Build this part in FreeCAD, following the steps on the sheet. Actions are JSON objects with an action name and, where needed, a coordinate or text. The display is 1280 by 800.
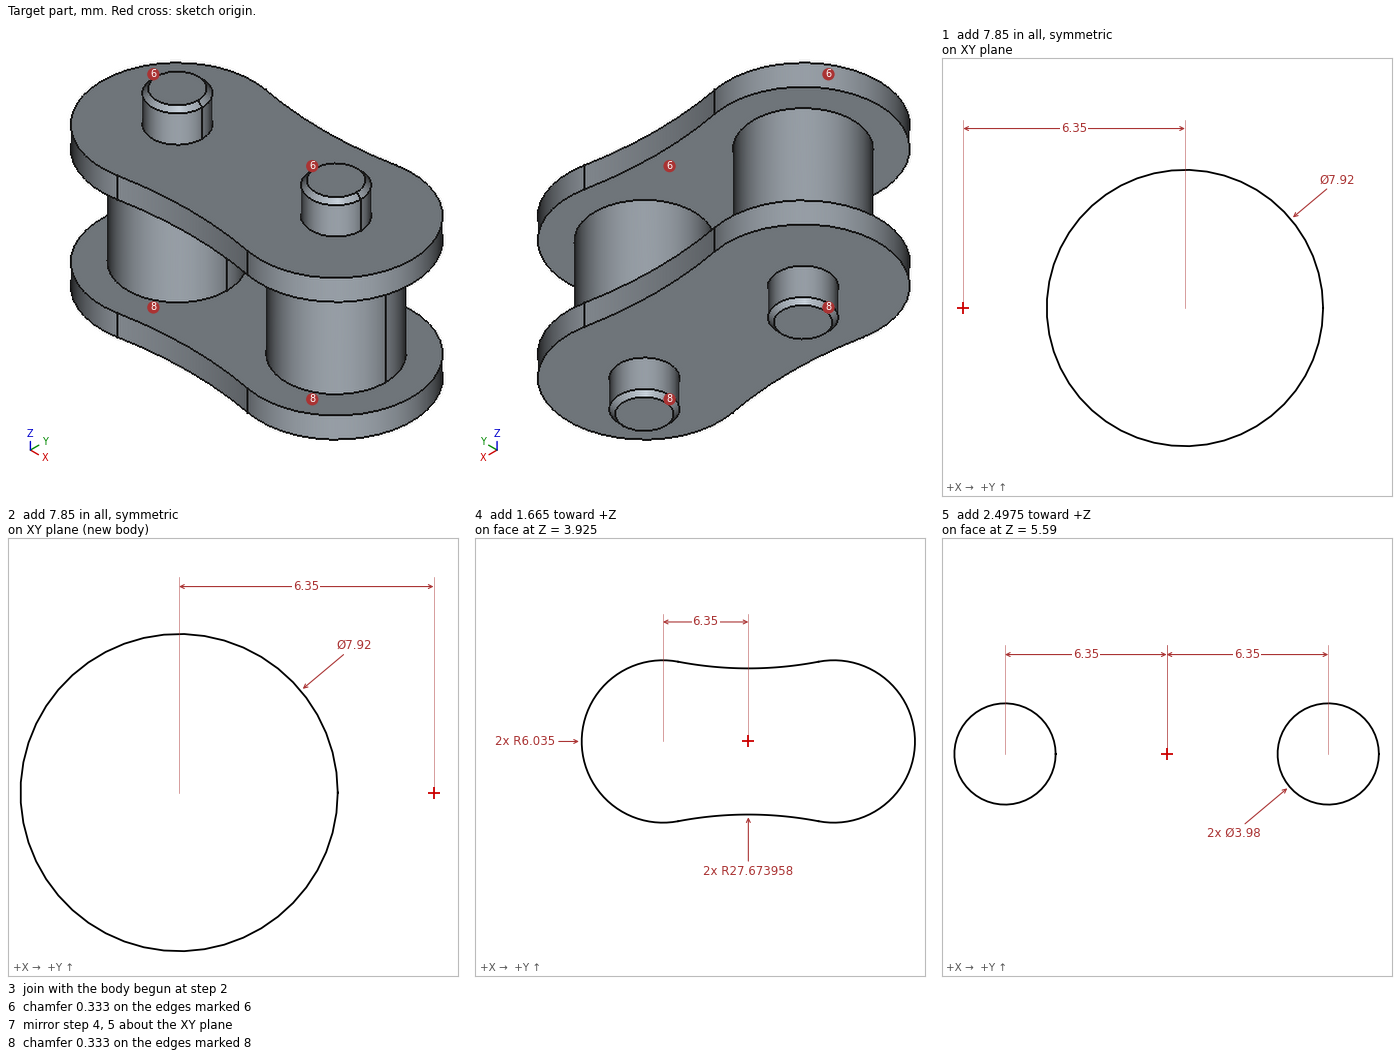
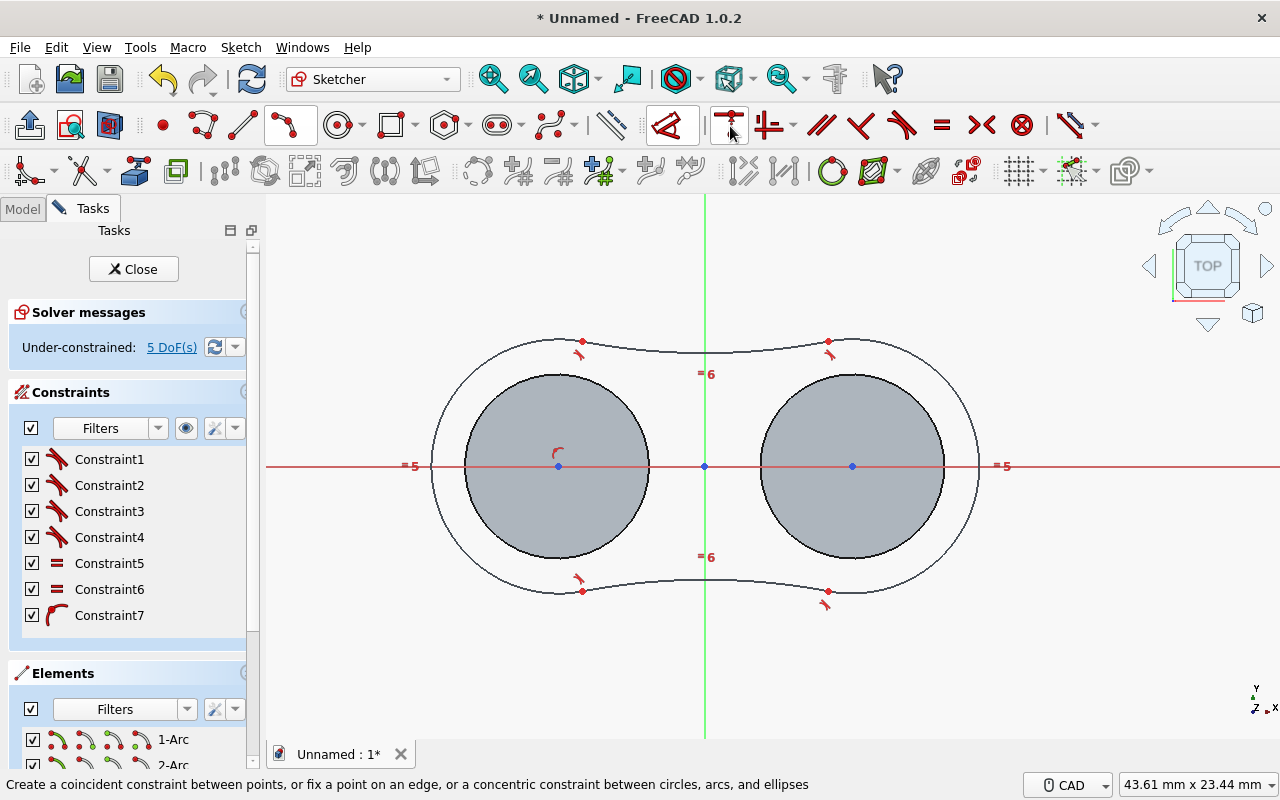
{"action": "scroll", "coordinate": [704, 282], "scroll_direction": "down", "scroll_amount": 5}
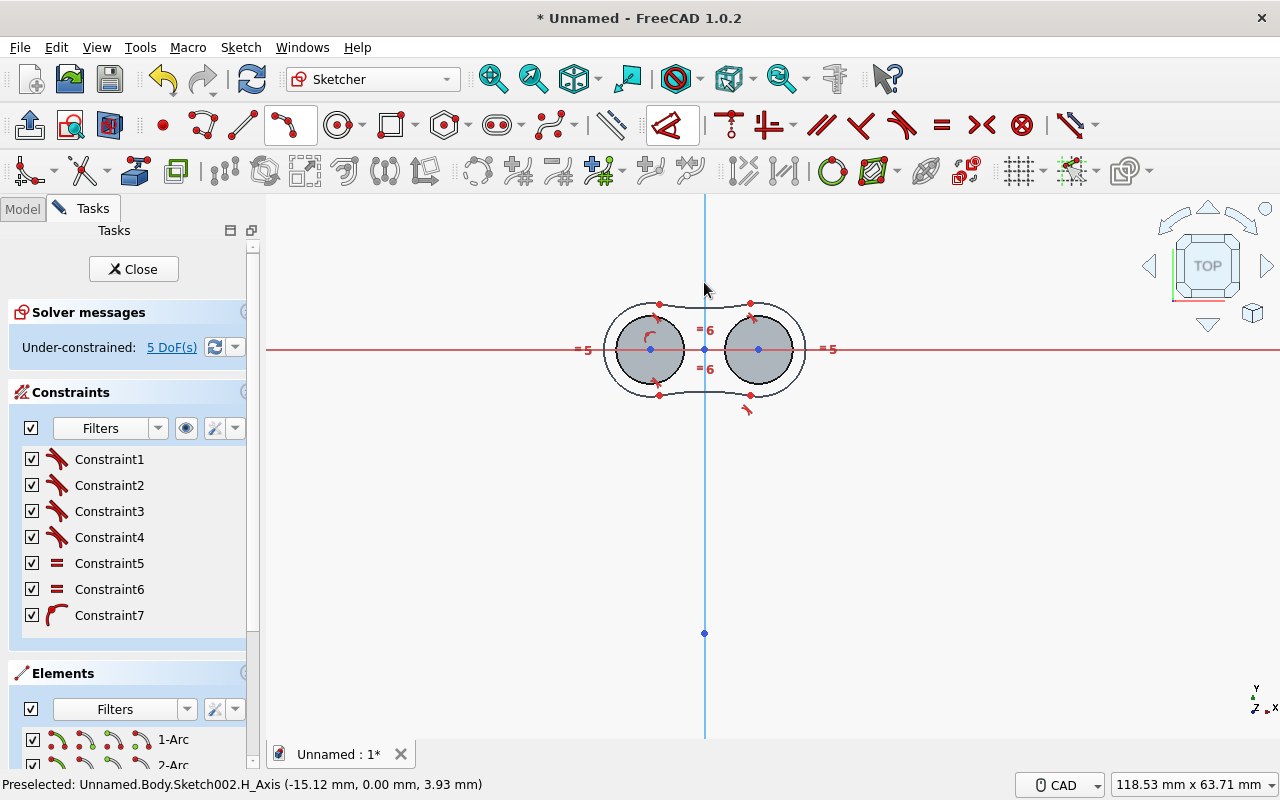
{"action": "left_click", "coordinate": [705, 634]}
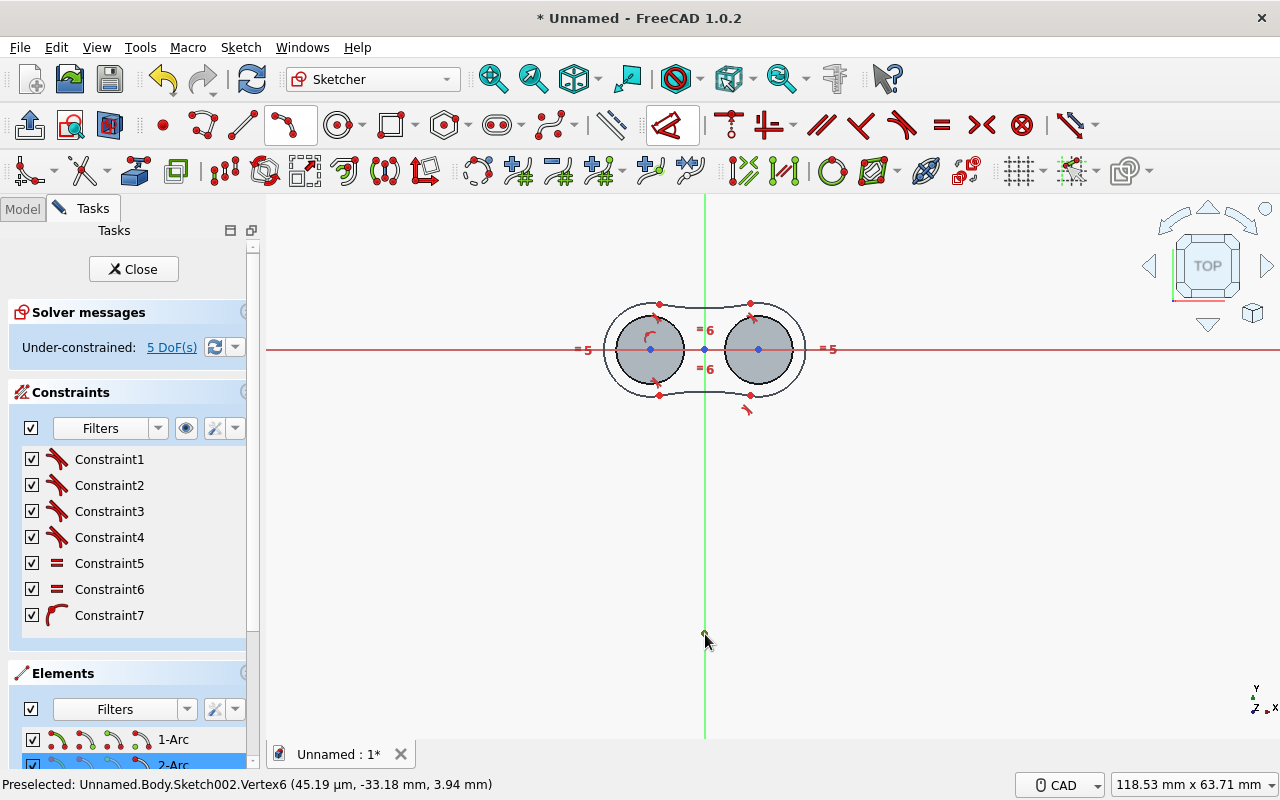
{"action": "left_click", "coordinate": [705, 676]}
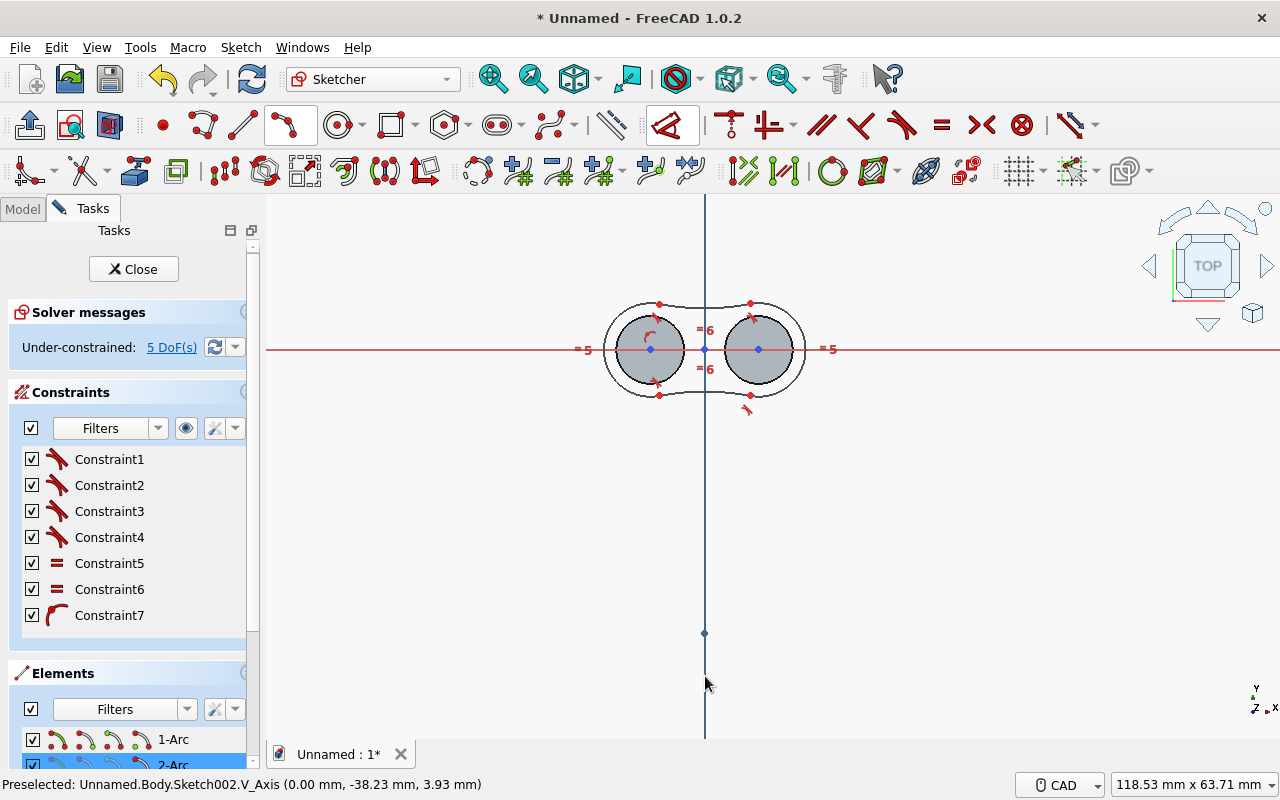
{"action": "key", "text": "c"}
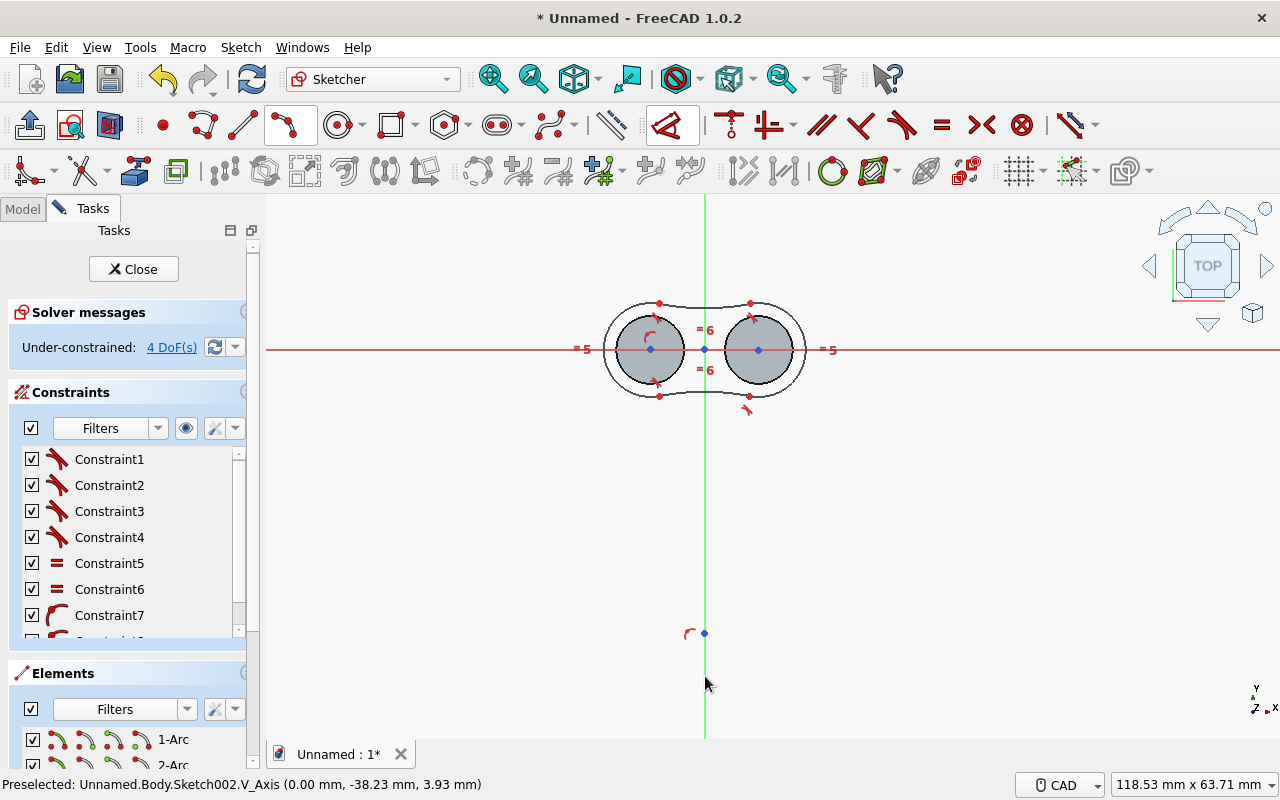
{"action": "left_click", "coordinate": [759, 350]}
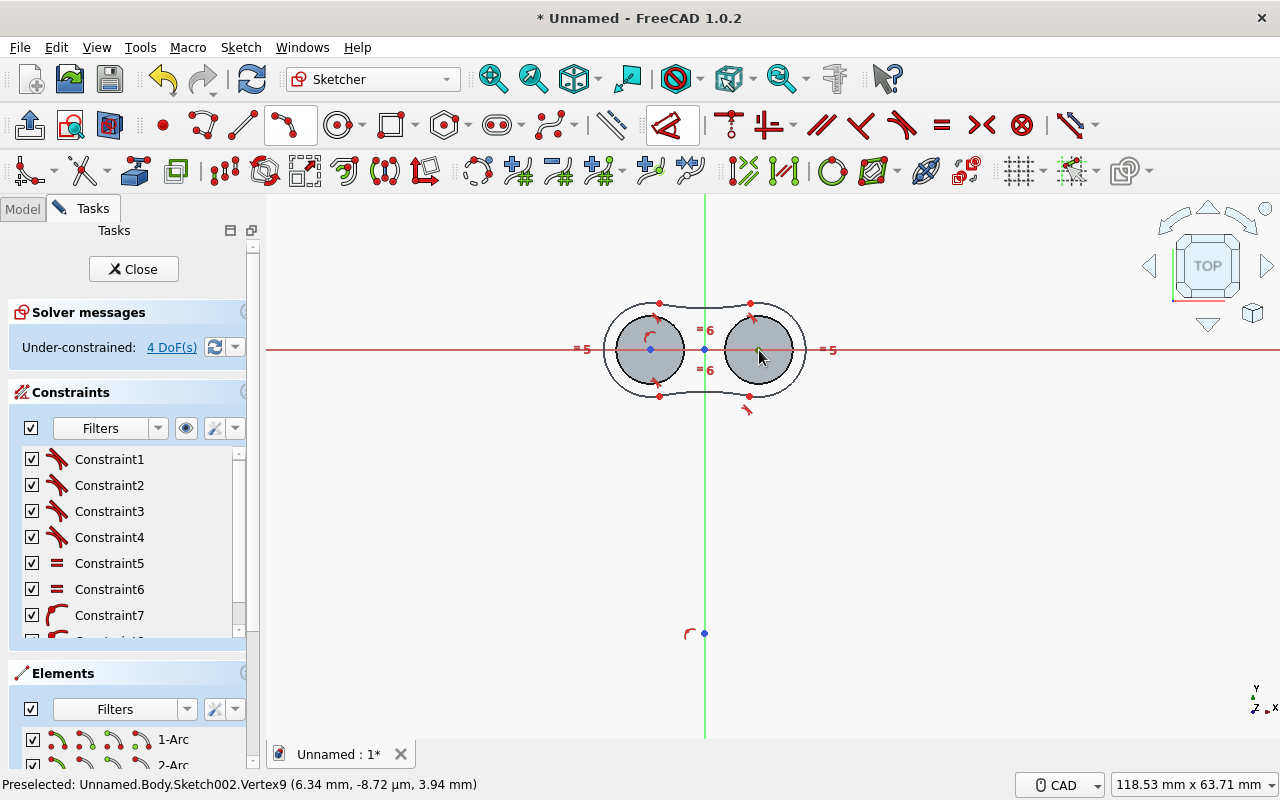
{"action": "left_click", "coordinate": [353, 350]}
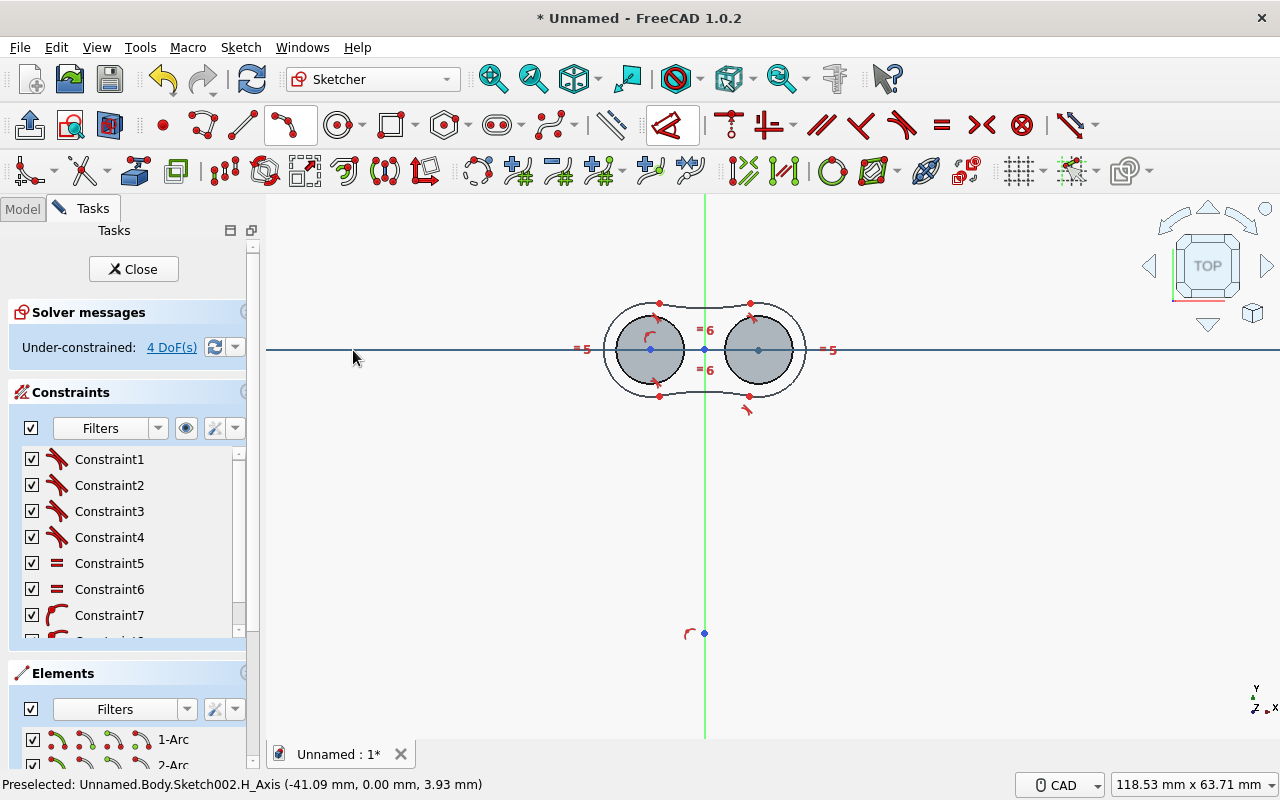
{"action": "left_click", "coordinate": [730, 126]}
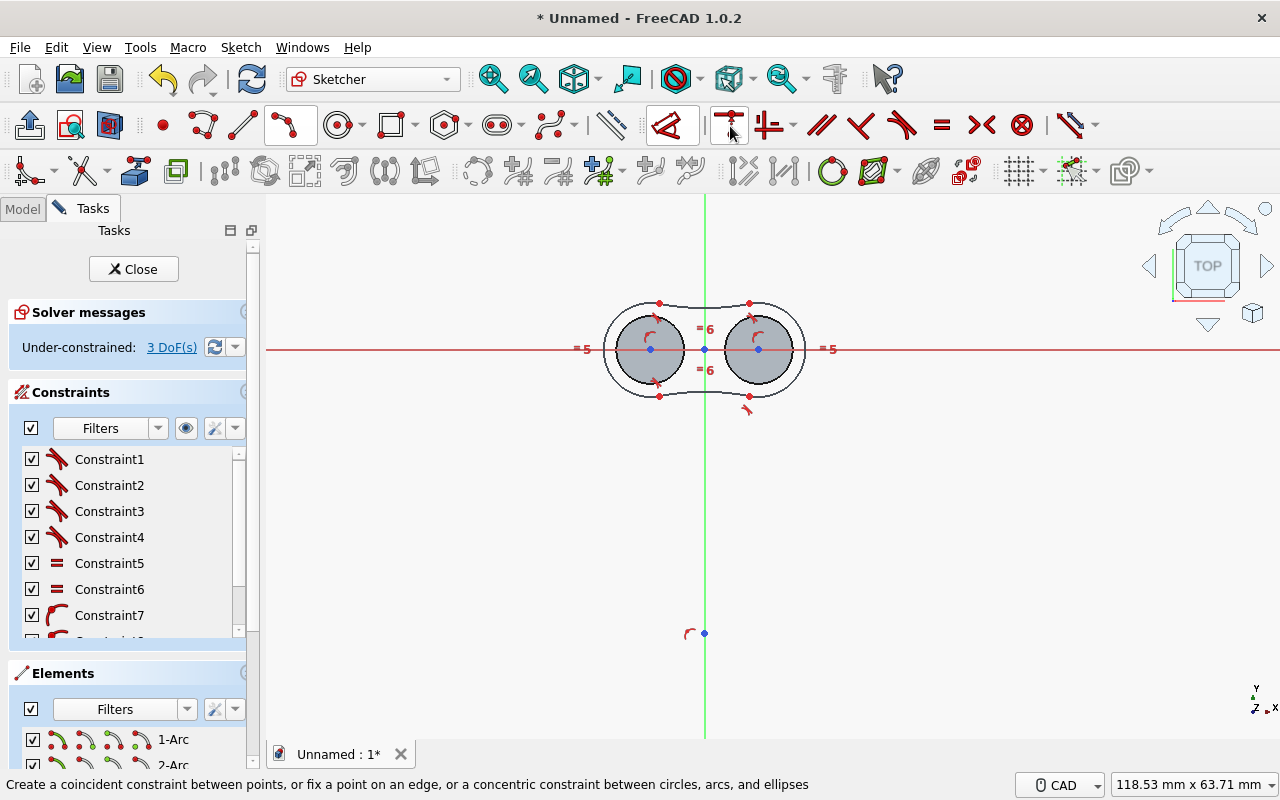
{"action": "left_click", "coordinate": [615, 320]}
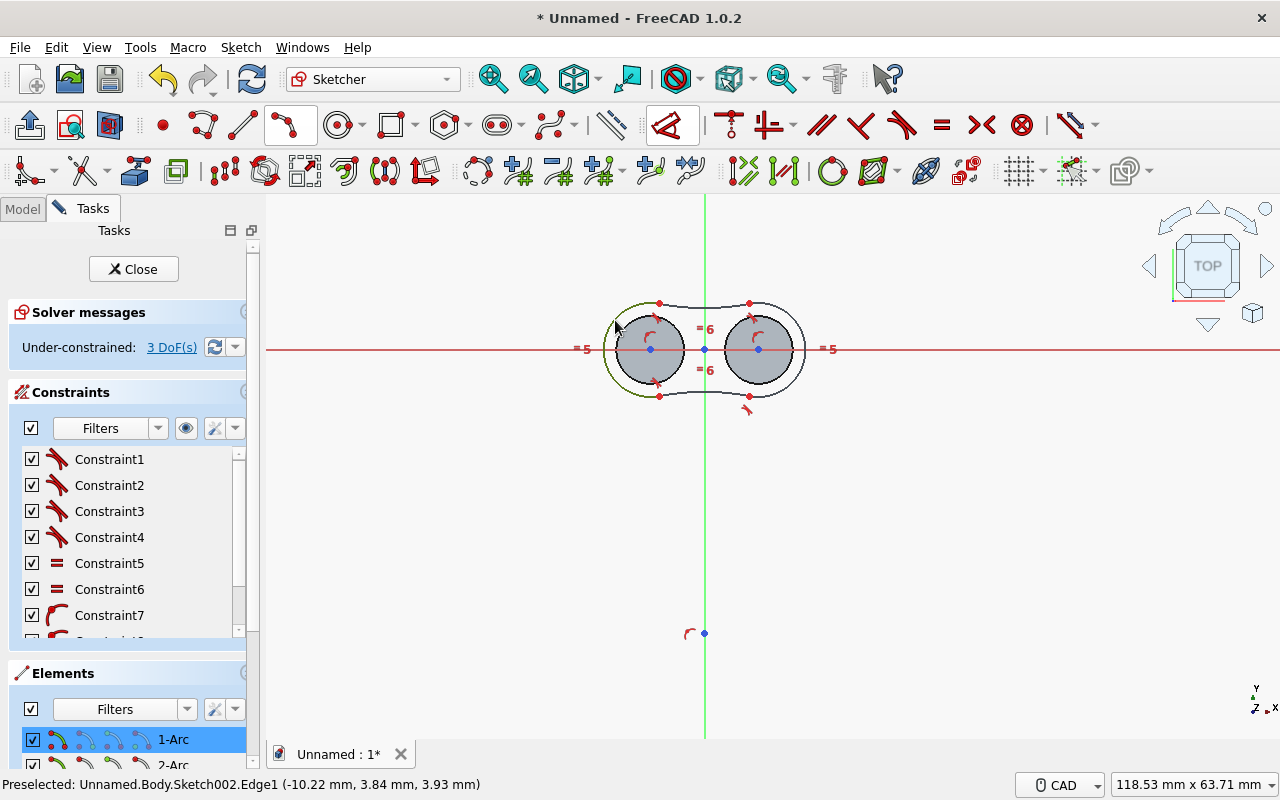
{"action": "key", "text": "k r"}